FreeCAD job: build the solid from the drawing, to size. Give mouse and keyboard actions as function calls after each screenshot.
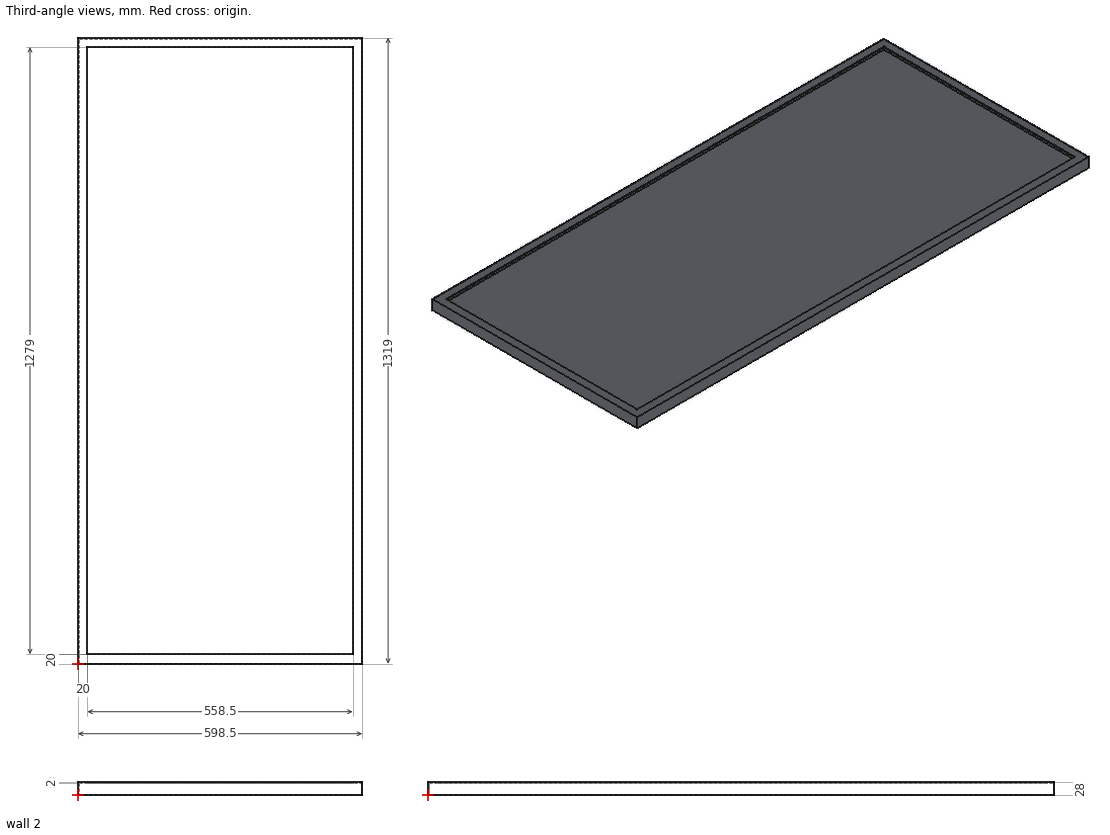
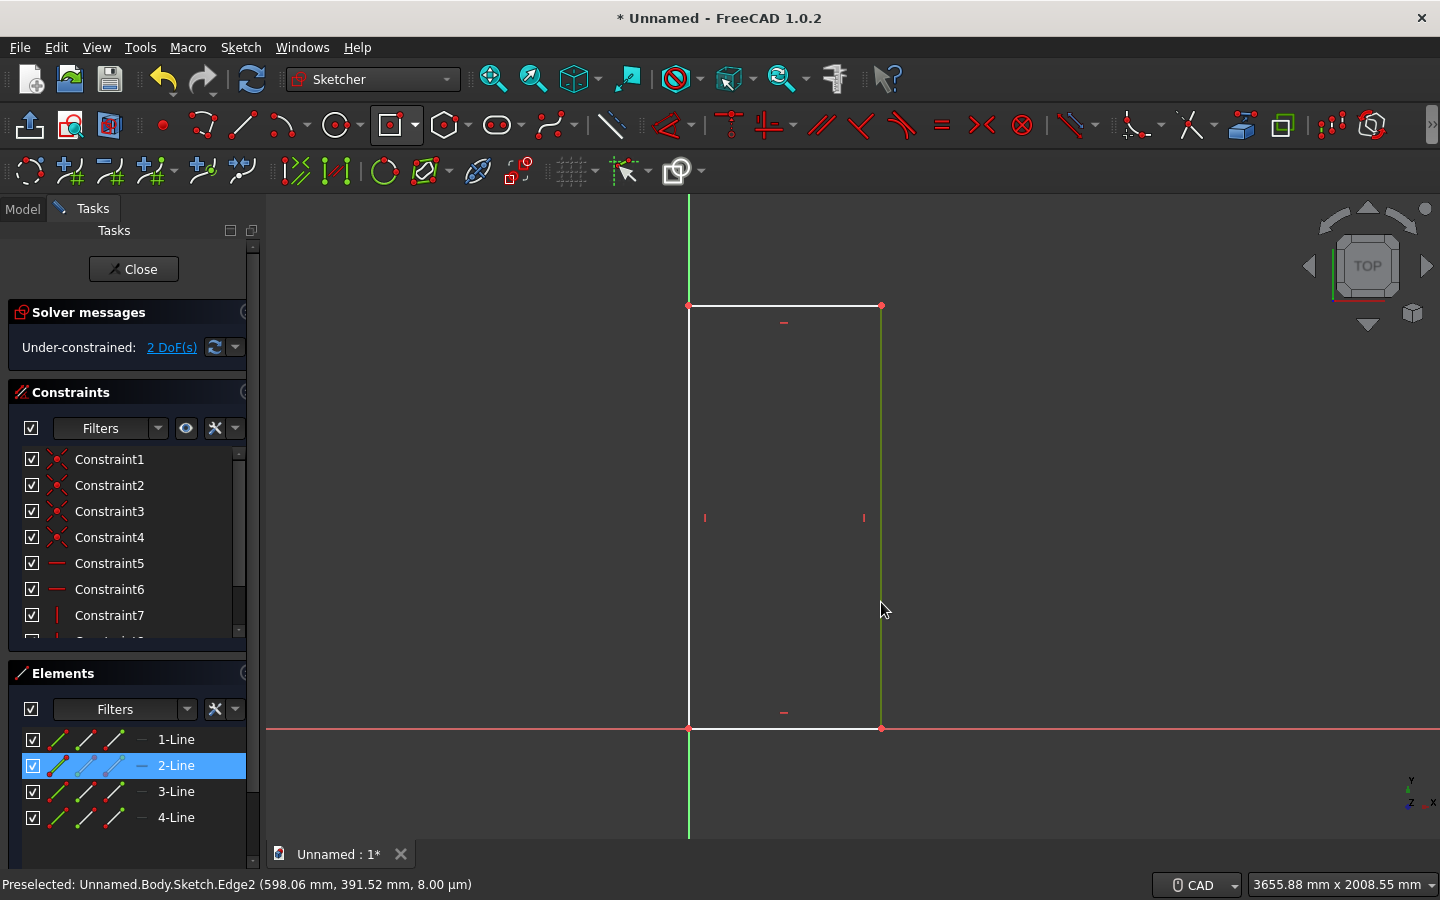
key(i)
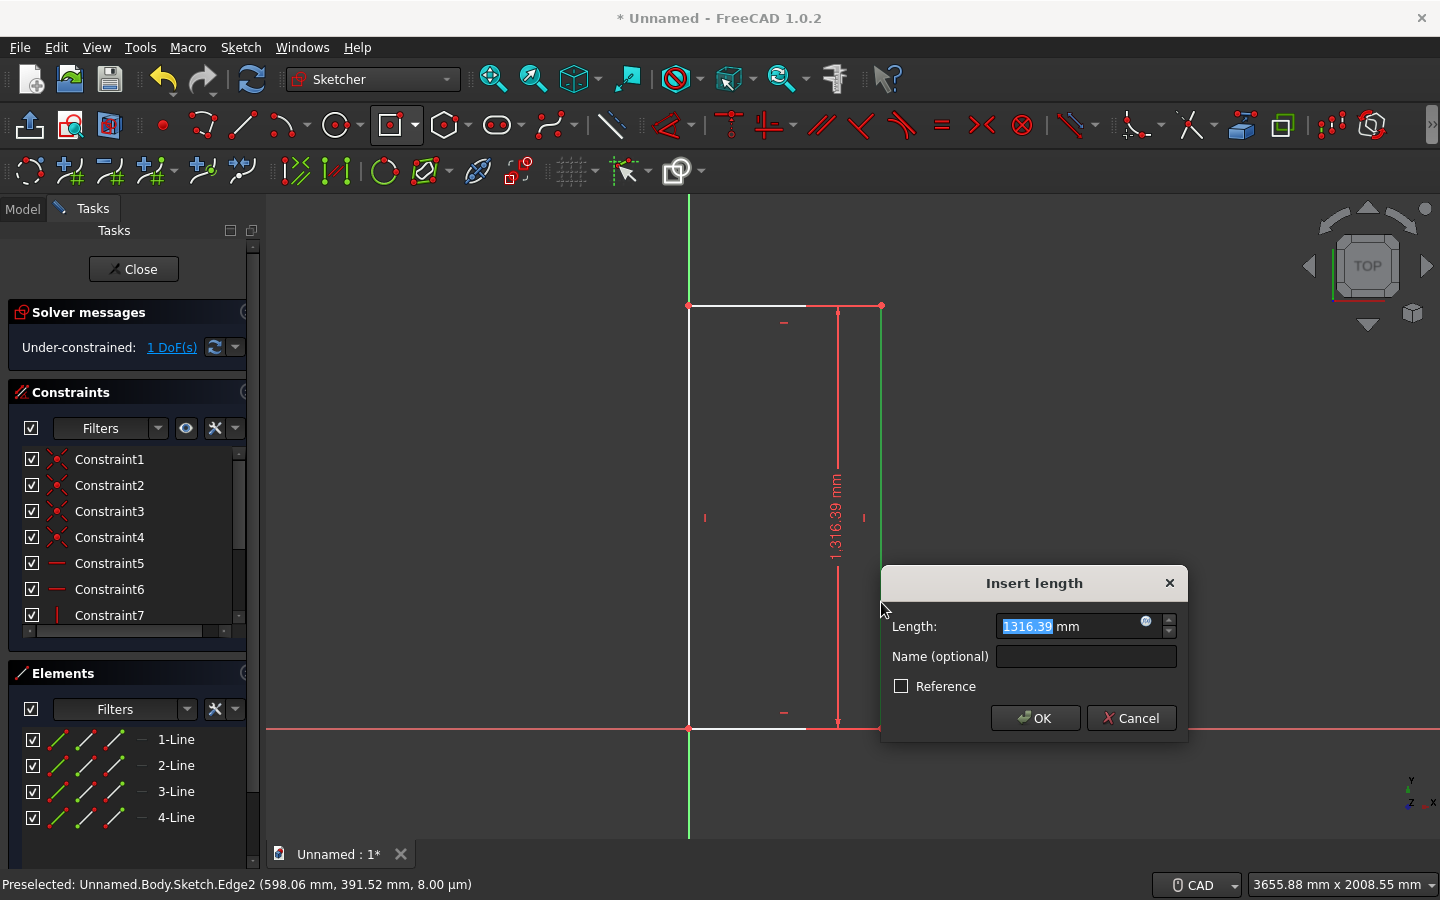
text(1319)
key(Return)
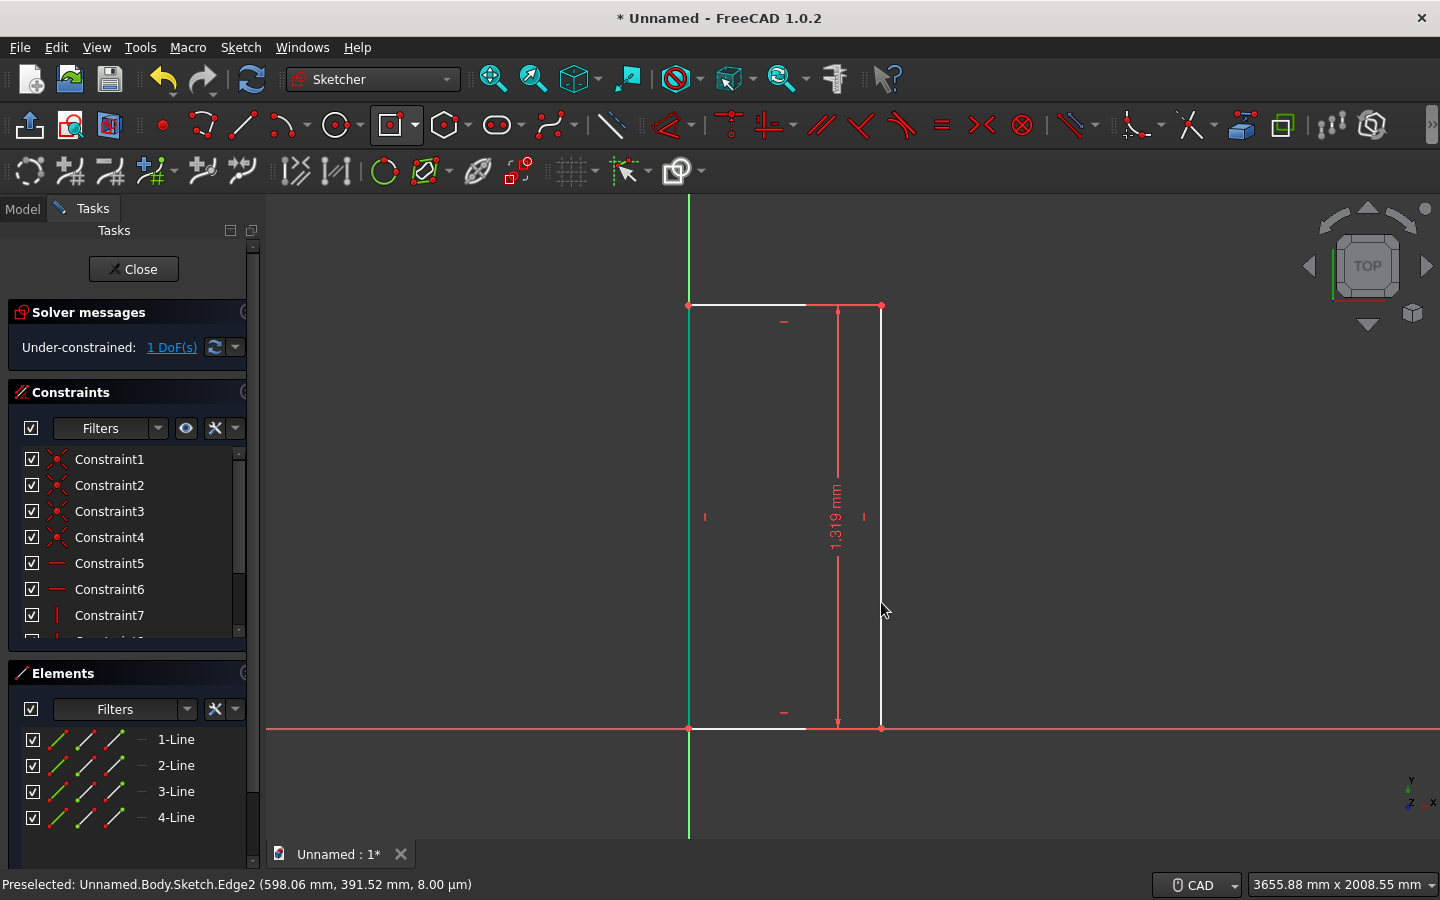
click(747, 729)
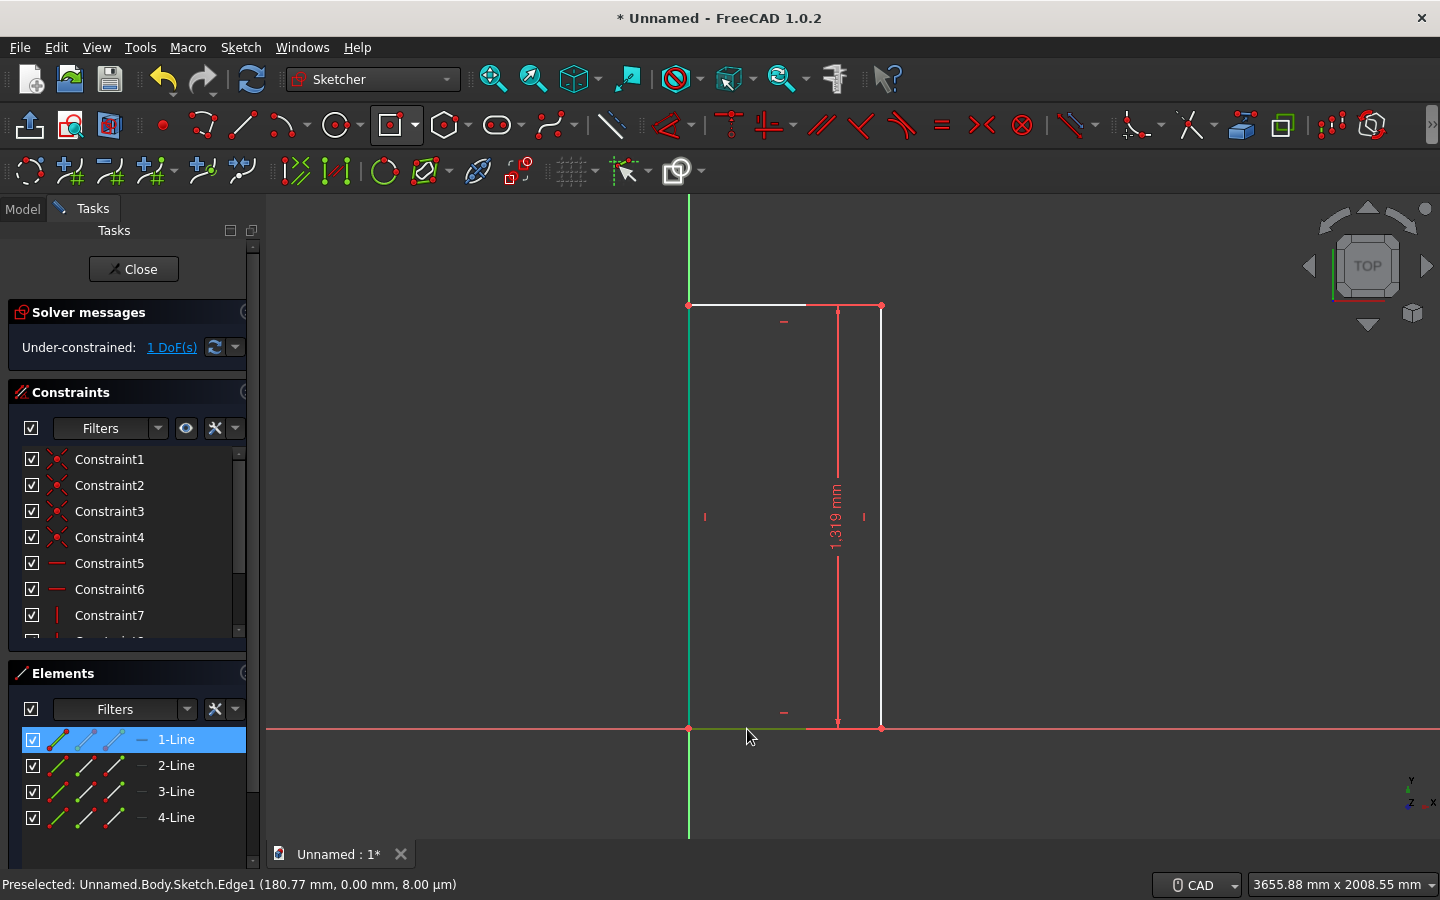
key(l)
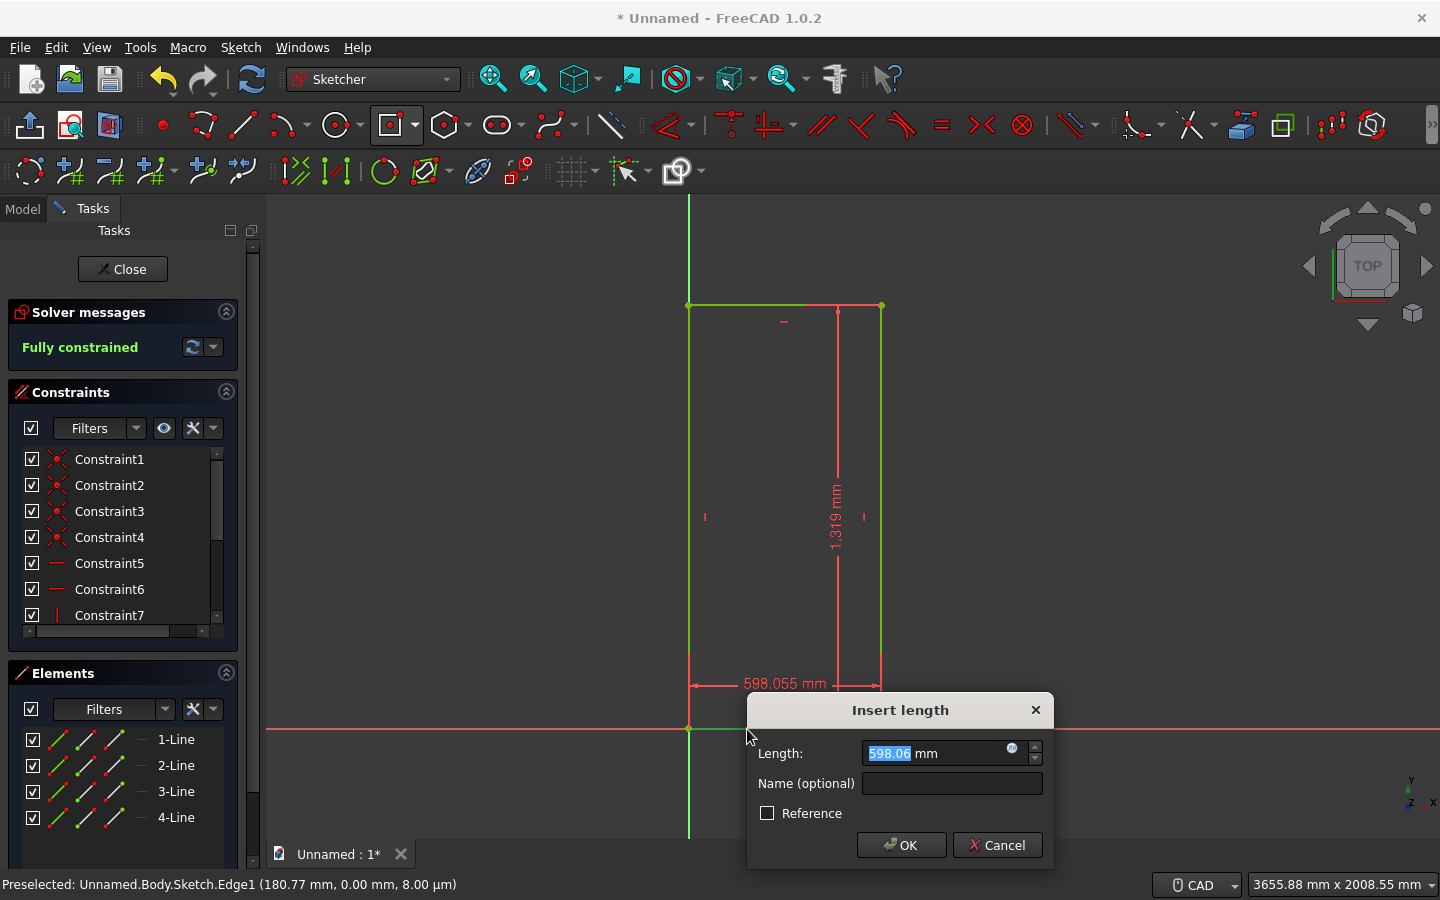
text(598.5)
key(Return)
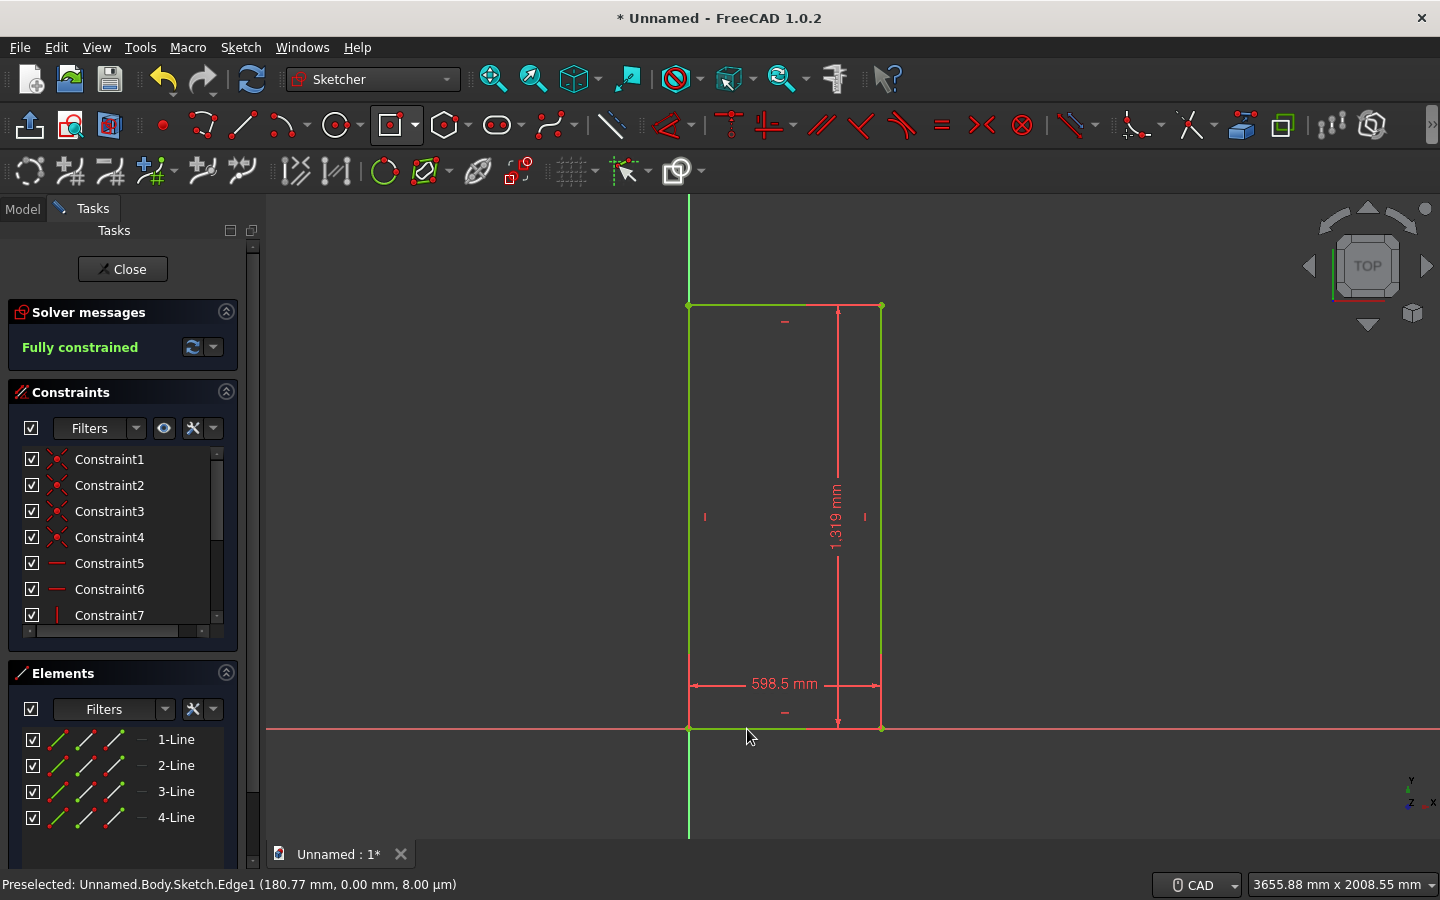
click(123, 269)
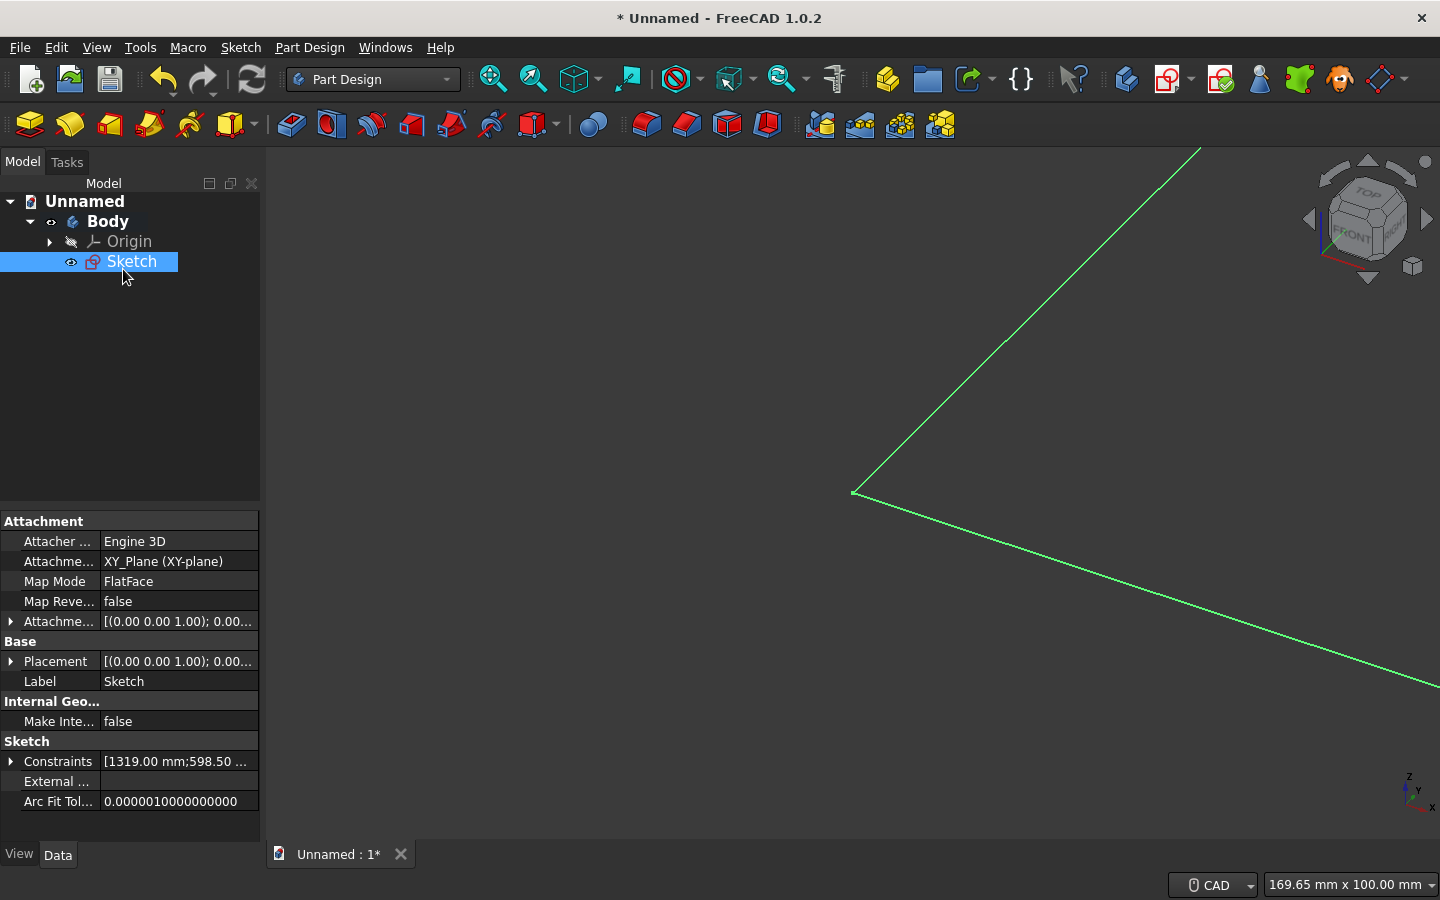
click(30, 124)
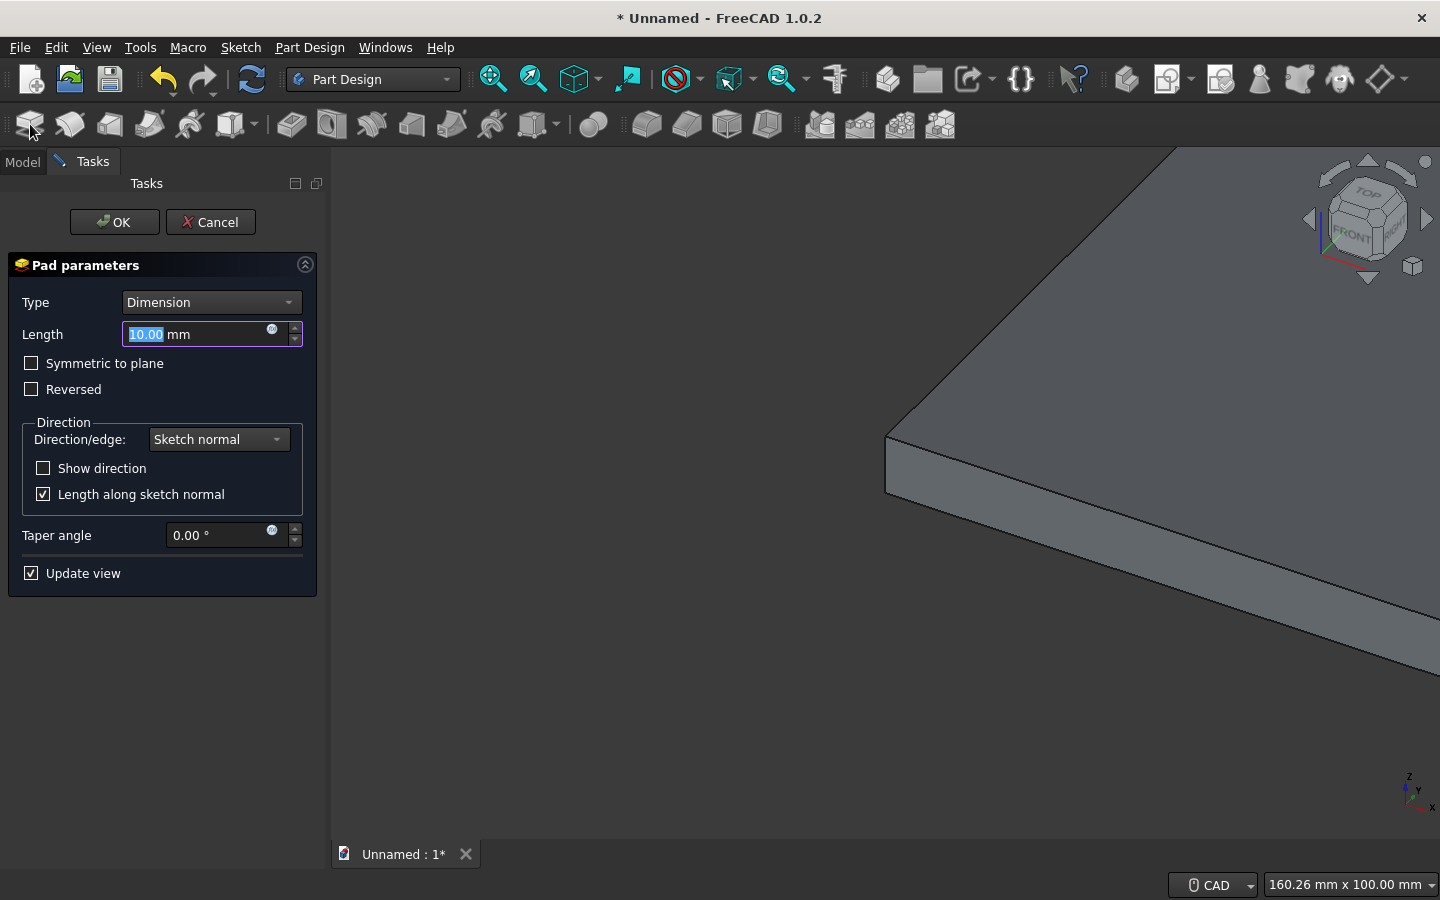
text(28)
key(Tab)